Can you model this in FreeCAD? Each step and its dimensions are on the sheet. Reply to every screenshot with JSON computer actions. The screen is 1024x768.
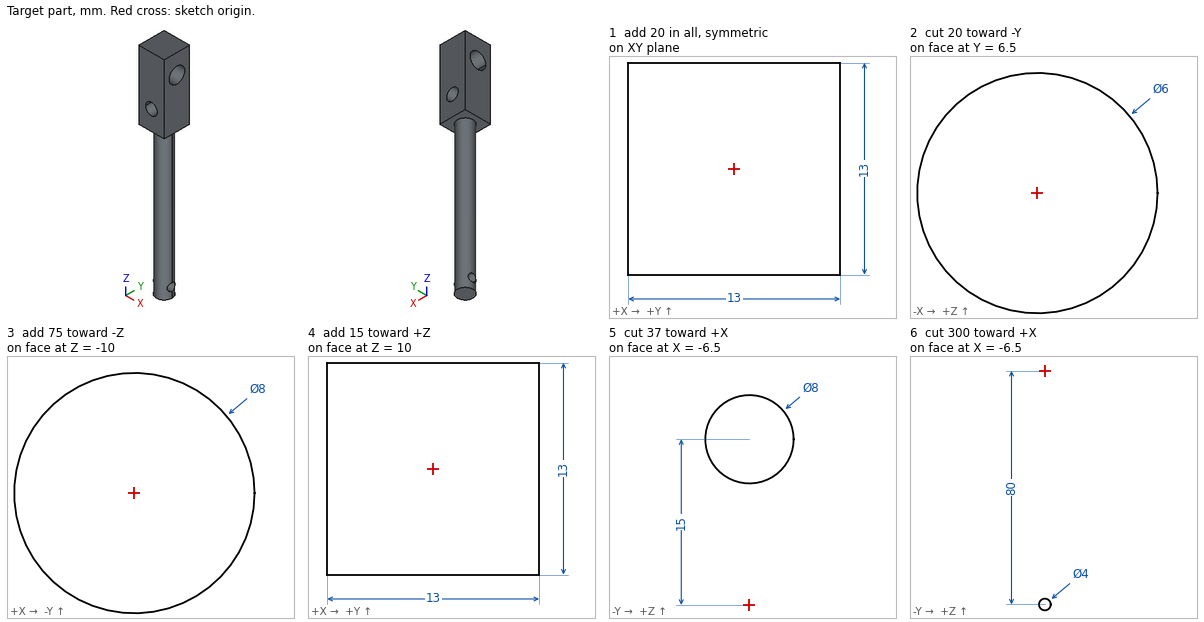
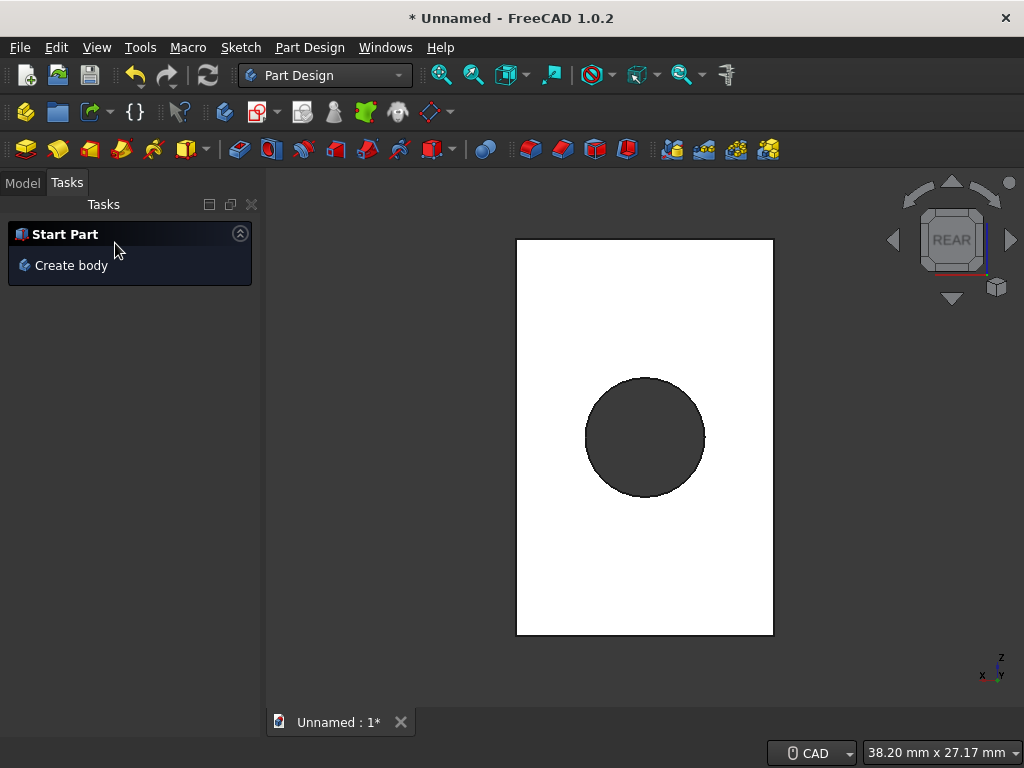
{"action": "key", "text": "5"}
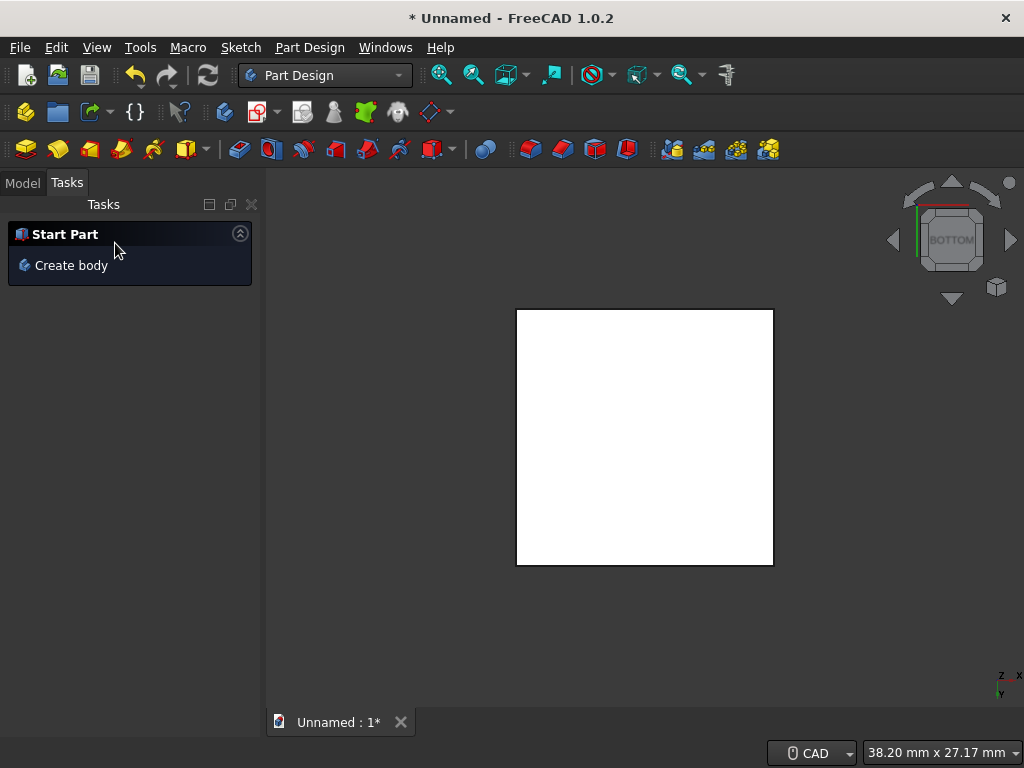
{"action": "left_click", "coordinate": [645, 437]}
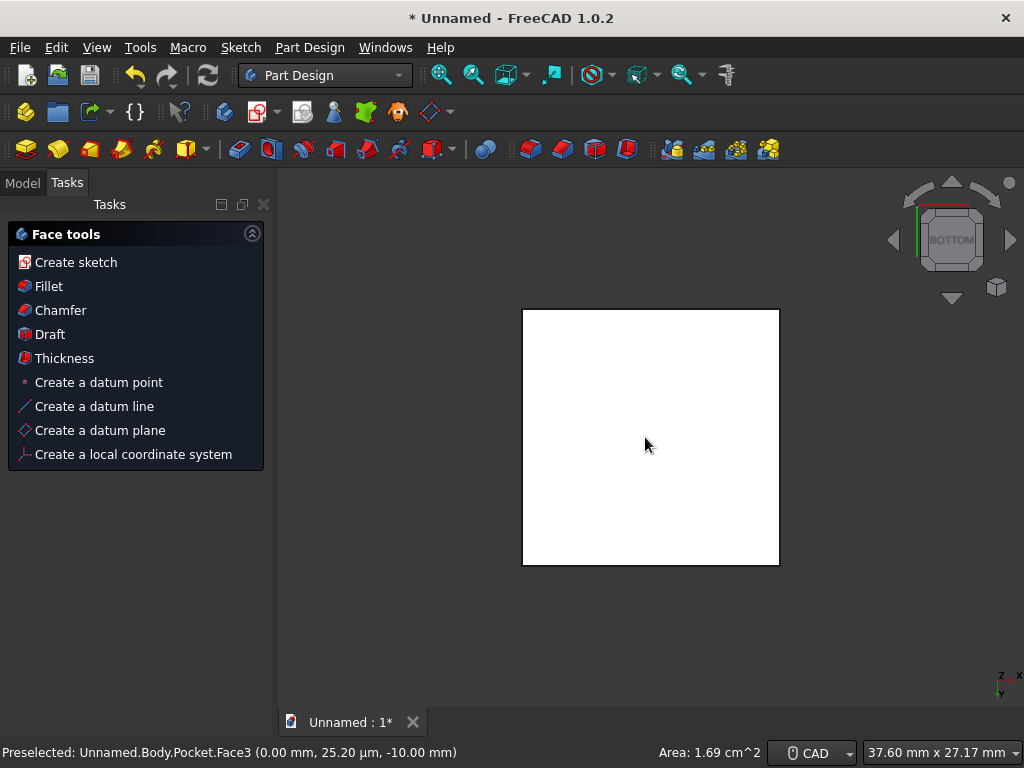
{"action": "left_click", "coordinate": [258, 112]}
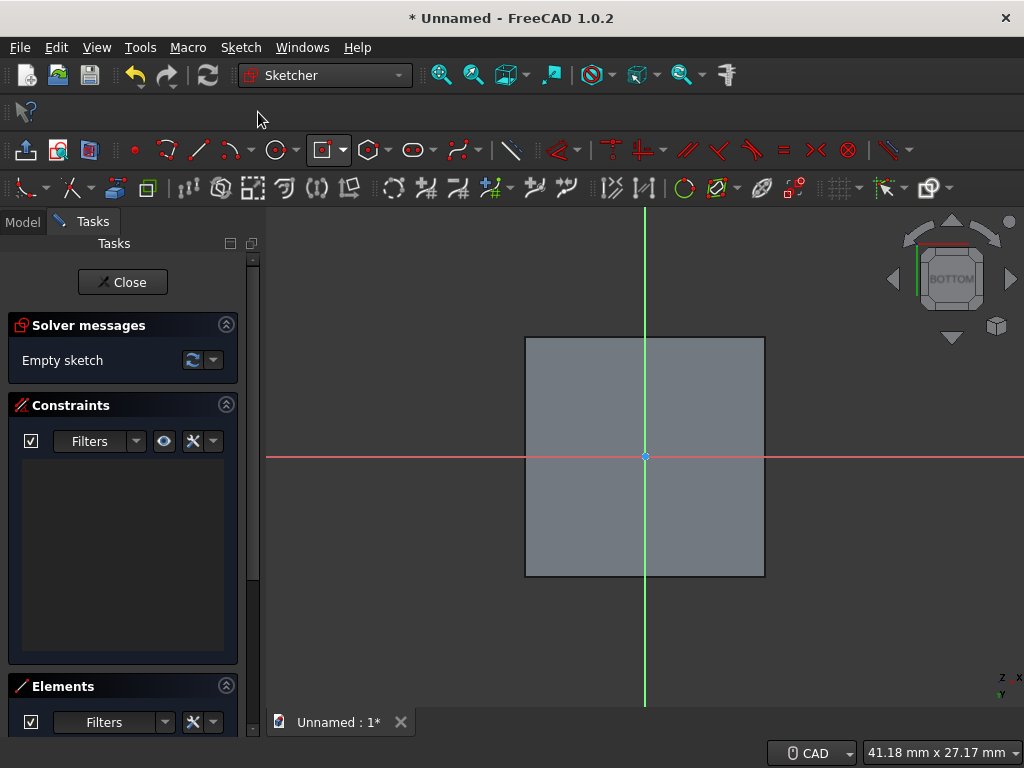
{"action": "scroll", "coordinate": [701, 457], "scroll_direction": "up", "scroll_amount": 4}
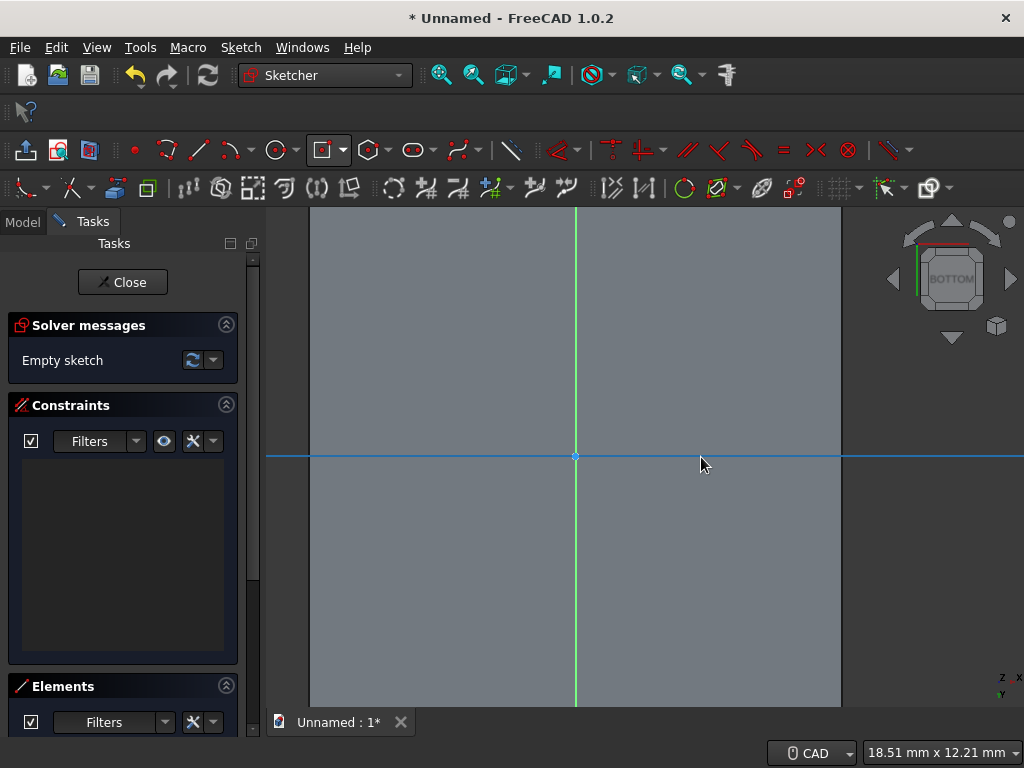
{"action": "left_click", "coordinate": [276, 150]}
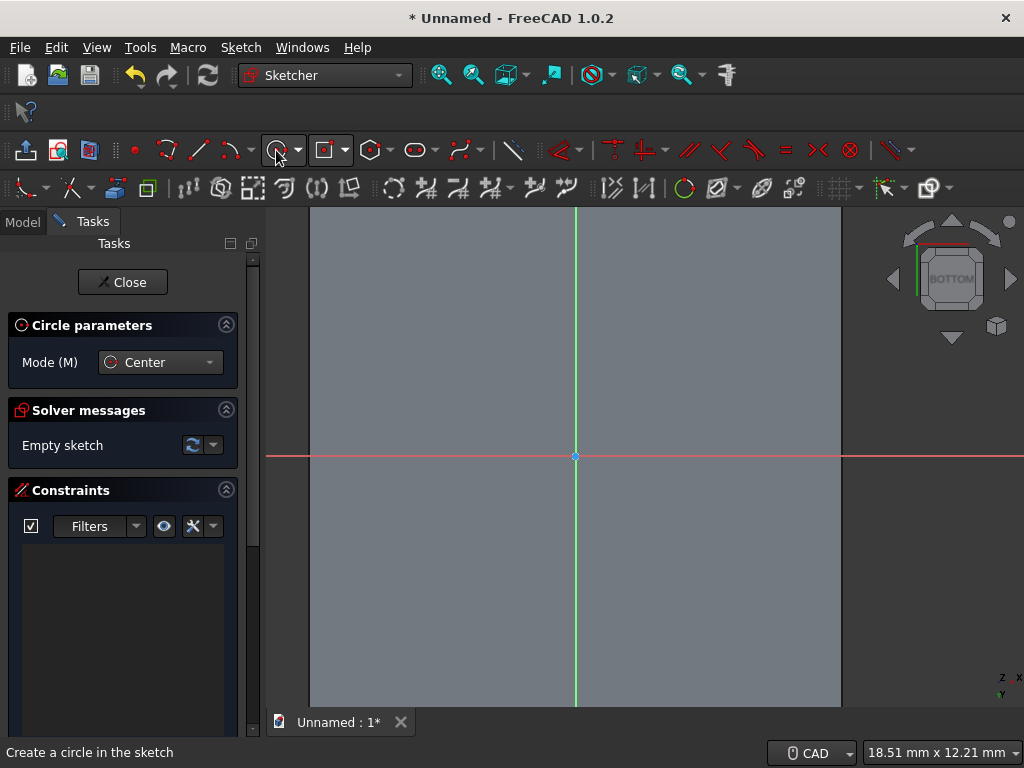
{"action": "left_click", "coordinate": [576, 456]}
{"action": "mouse_move", "coordinate": [692, 341]}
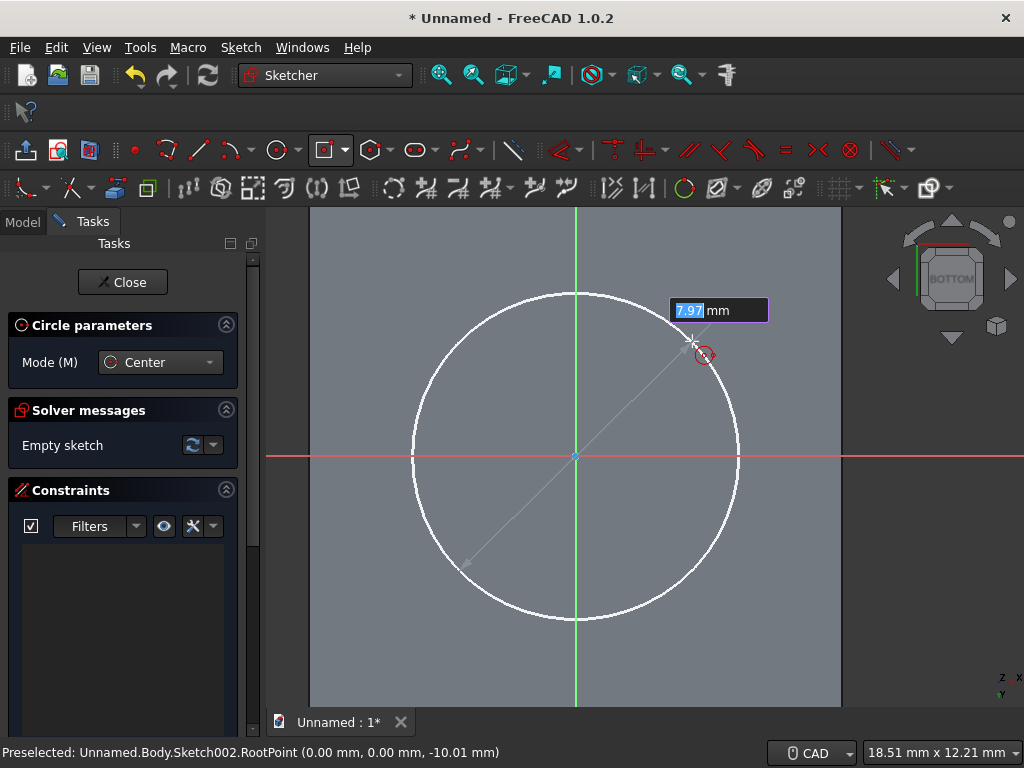
{"action": "type", "text": "8"}
{"action": "key", "text": "Return"}
{"action": "key", "text": "Escape"}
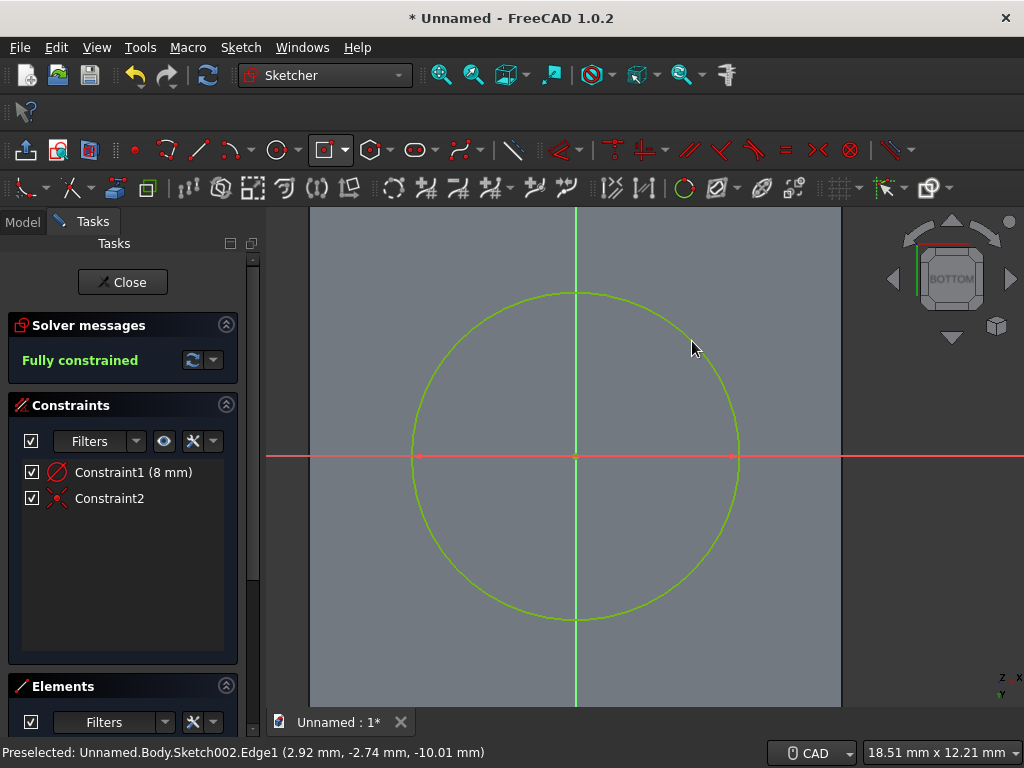
{"action": "left_click", "coordinate": [123, 282]}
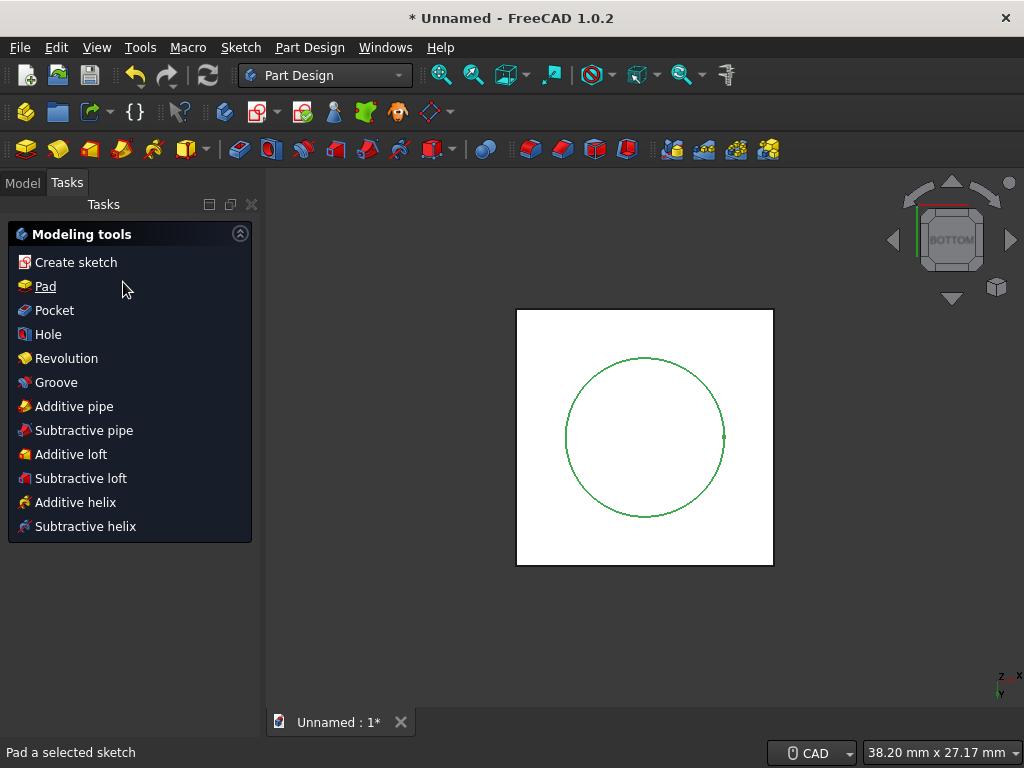
{"action": "left_click", "coordinate": [26, 150]}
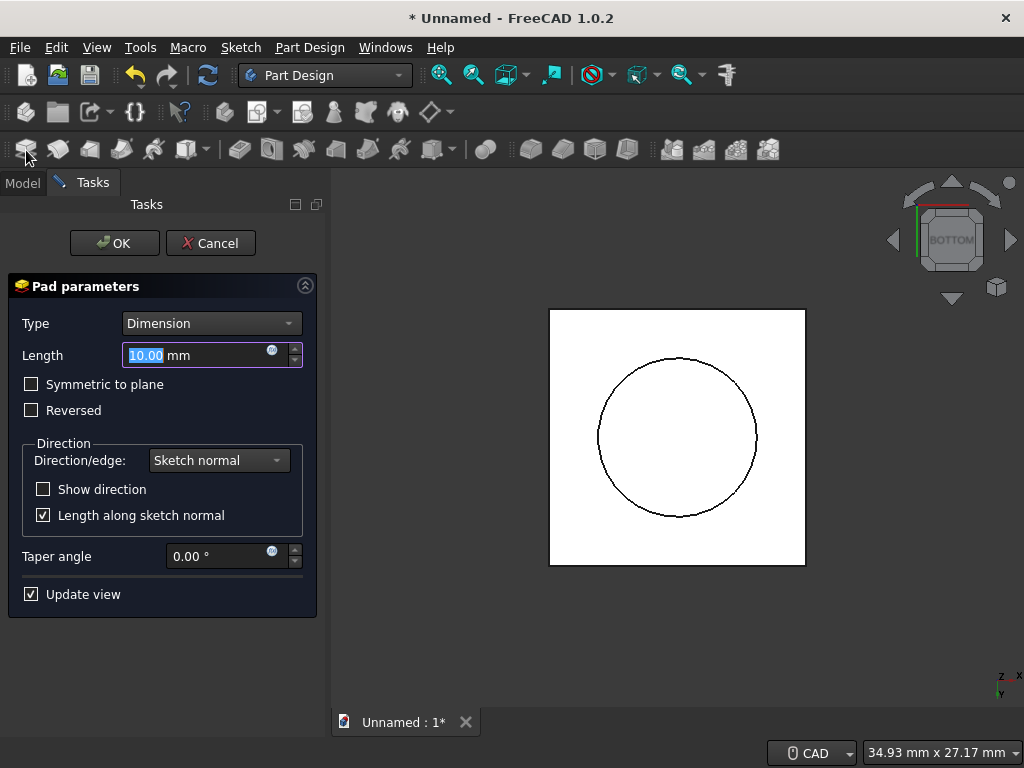
{"action": "type", "text": "75"}
{"action": "key", "text": "Tab"}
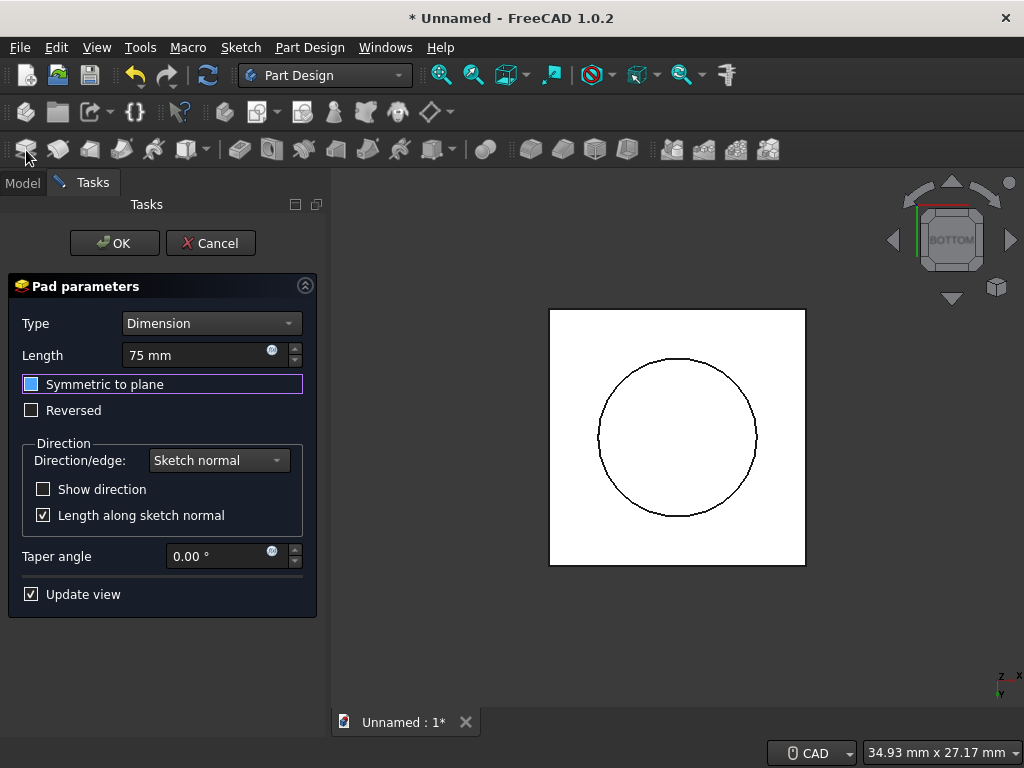
{"action": "left_click", "coordinate": [115, 243]}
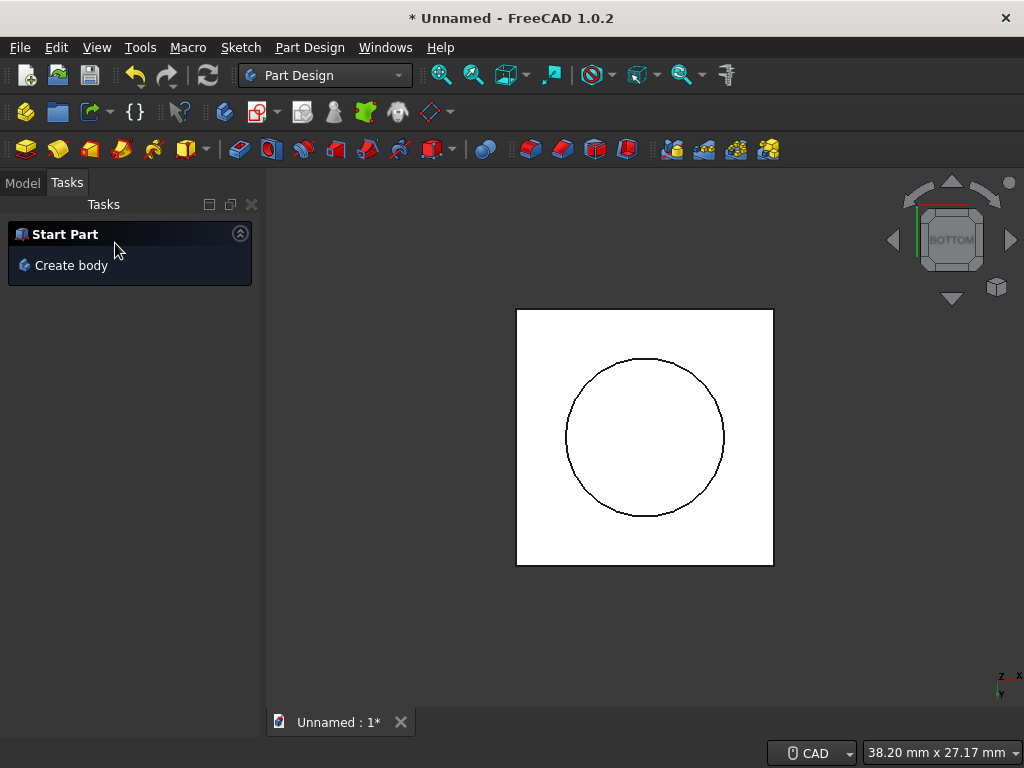
{"action": "key", "text": "0"}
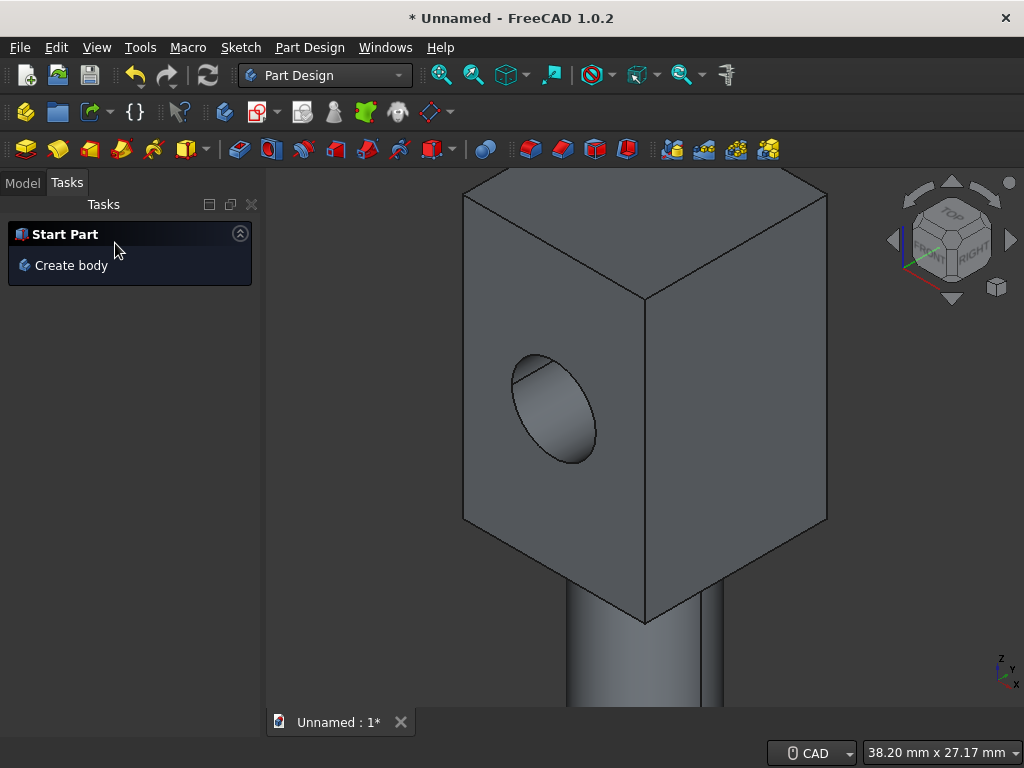
{"action": "left_click", "coordinate": [442, 76]}